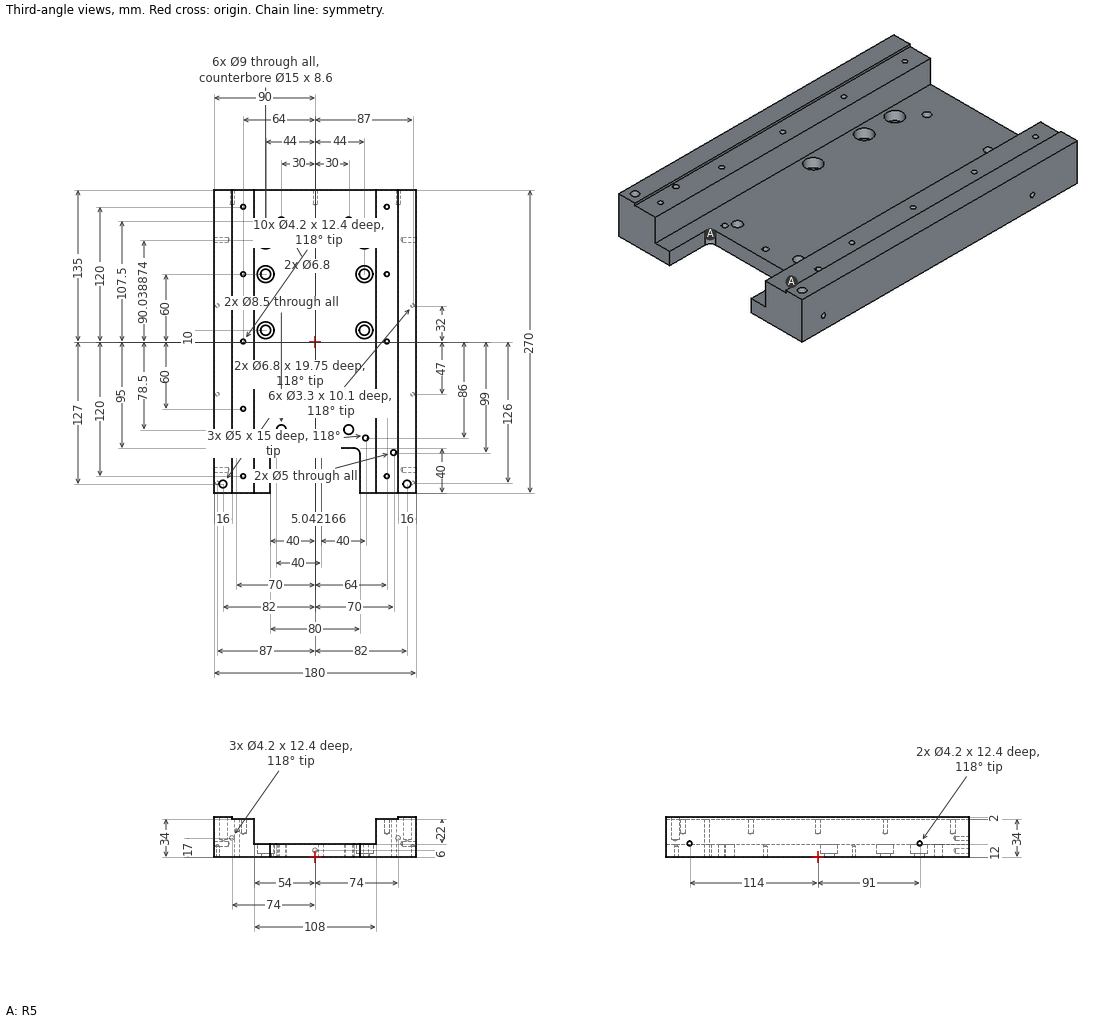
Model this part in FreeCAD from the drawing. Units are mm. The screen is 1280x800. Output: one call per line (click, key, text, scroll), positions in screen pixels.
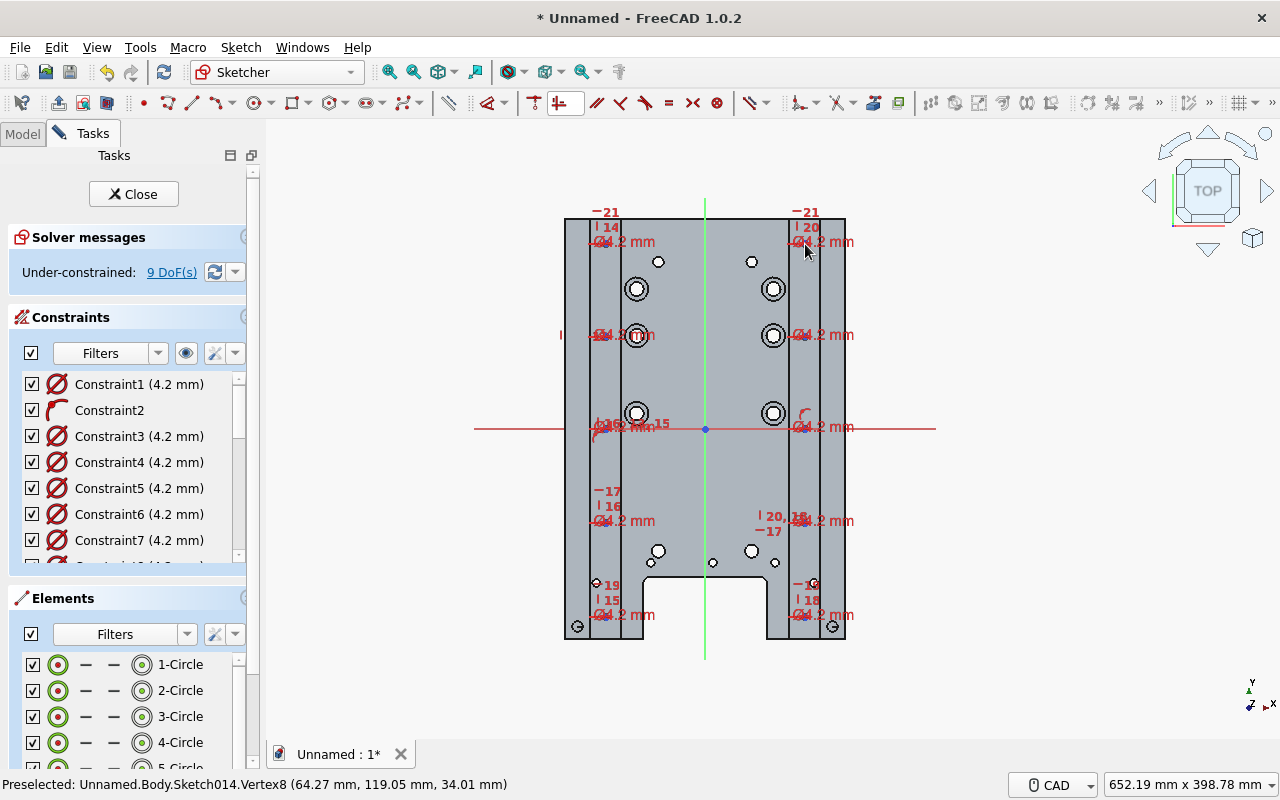
click(805, 244)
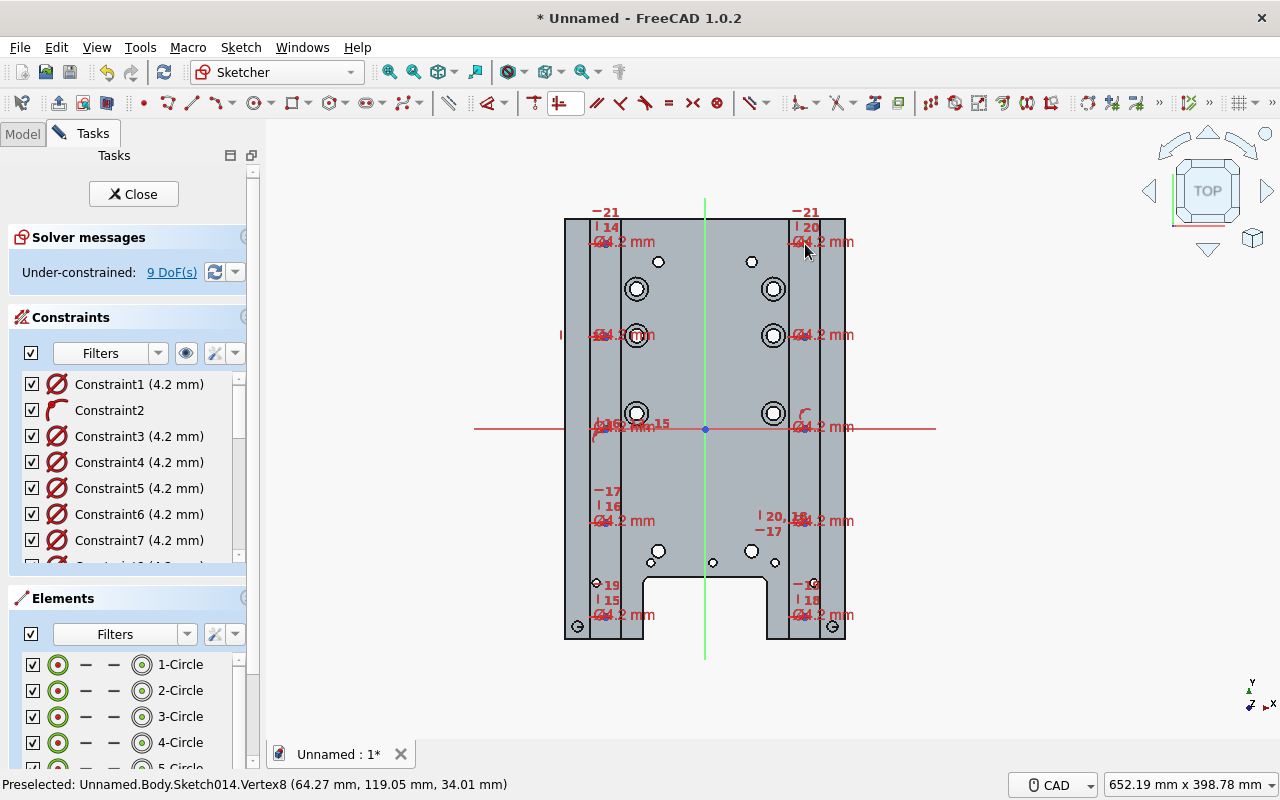
click(805, 337)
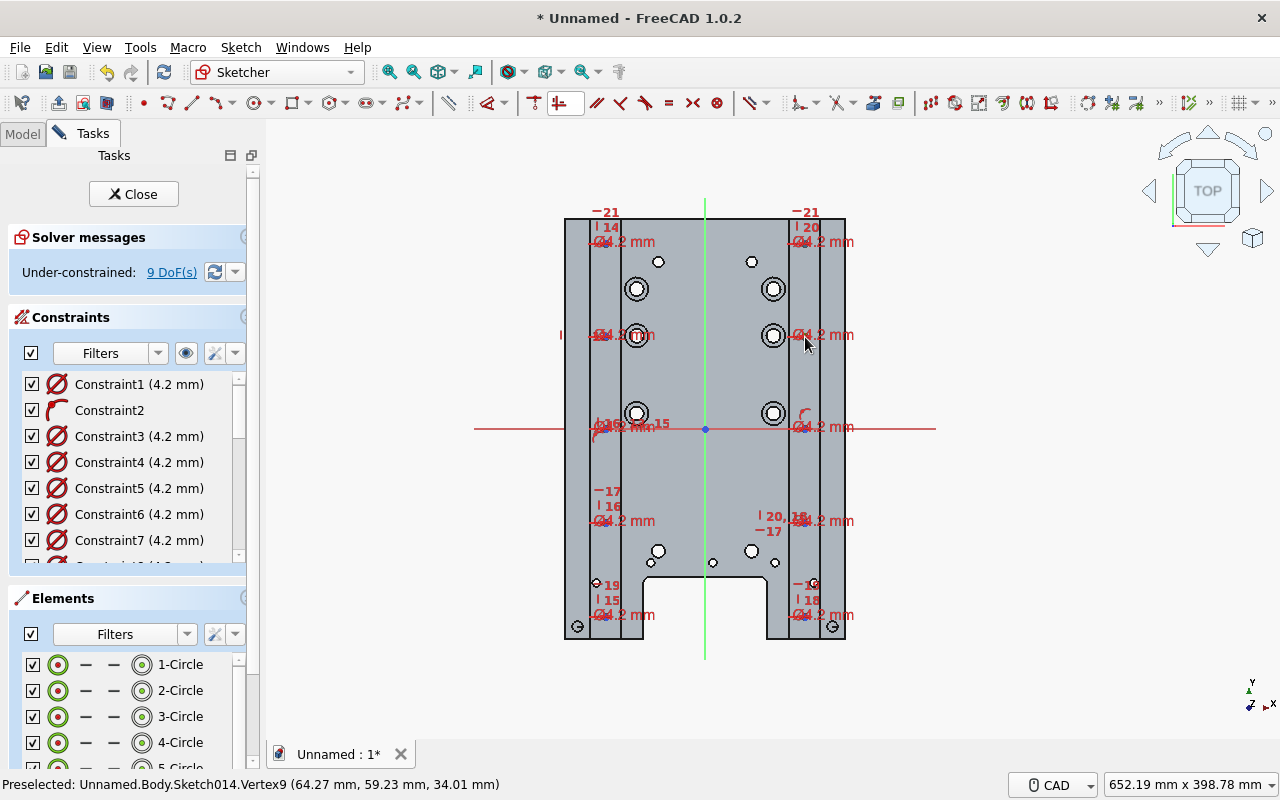
key(v)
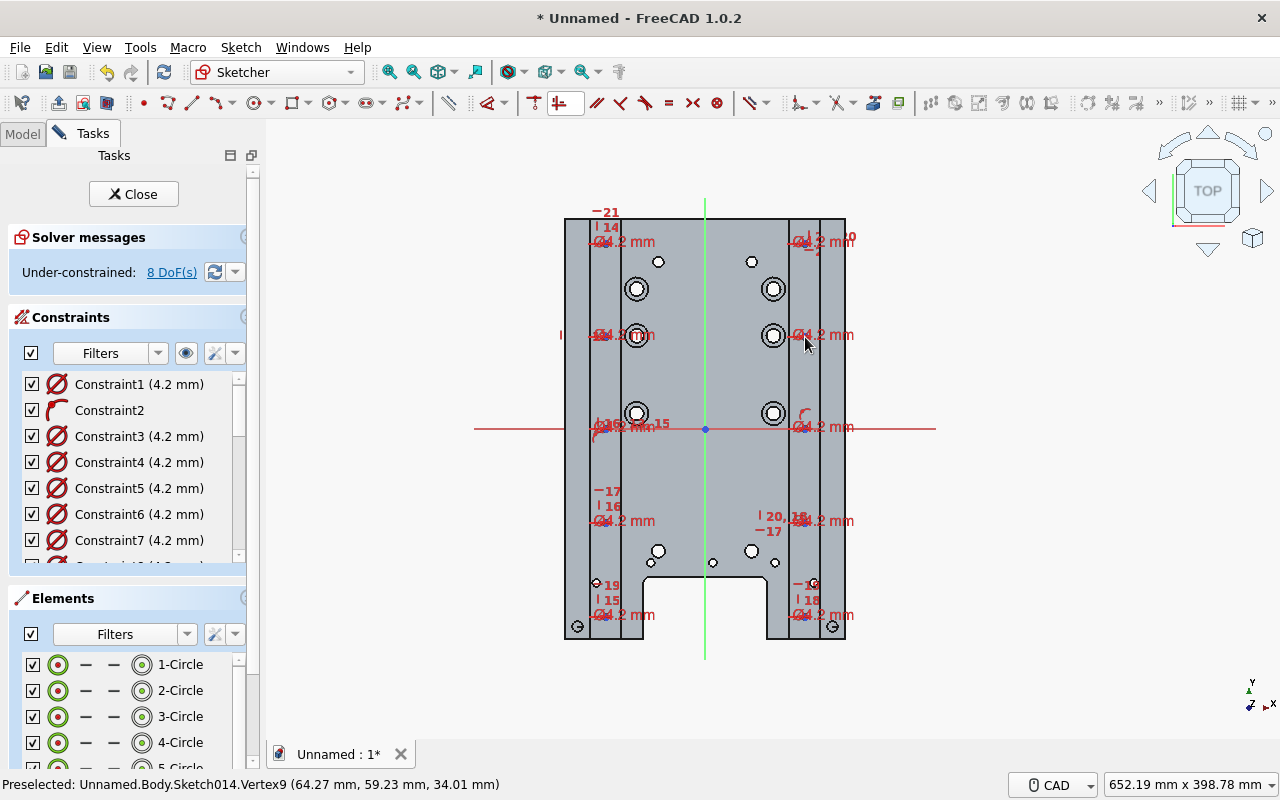
click(606, 337)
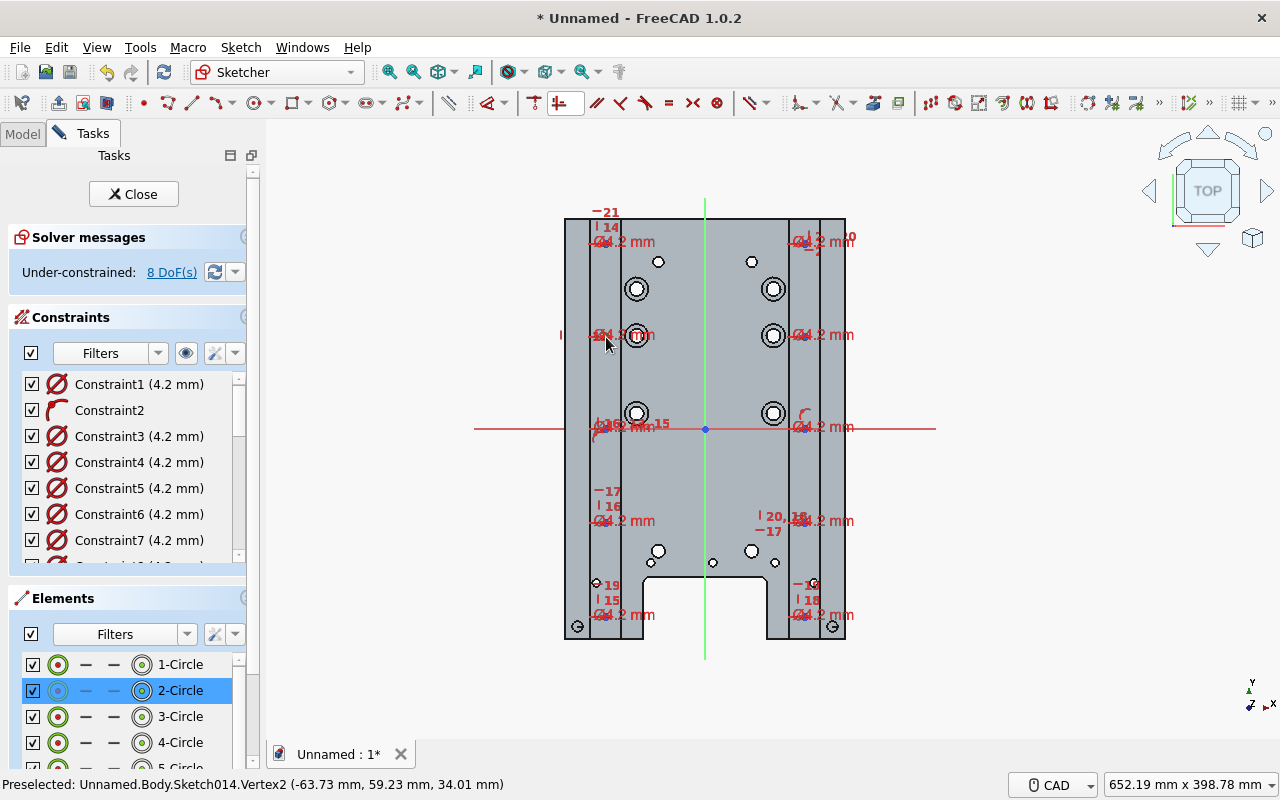
click(805, 337)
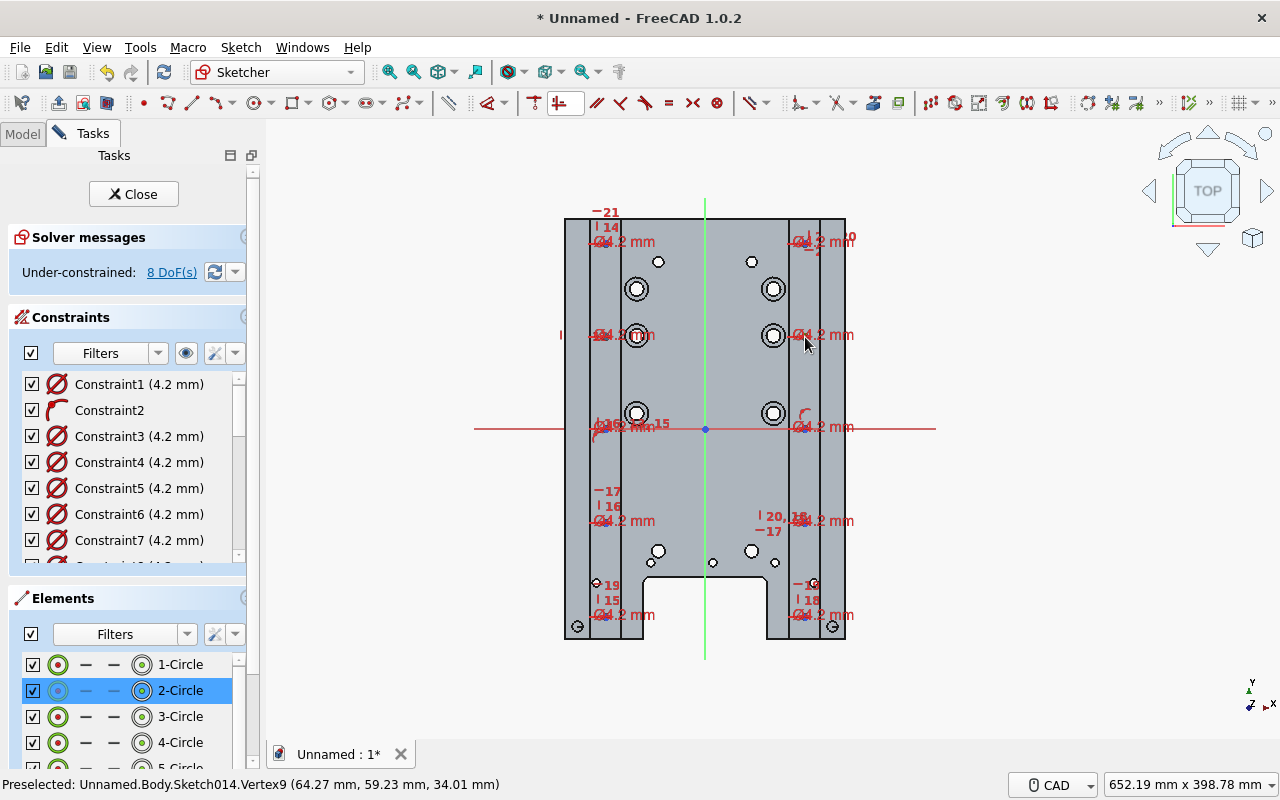
key(h)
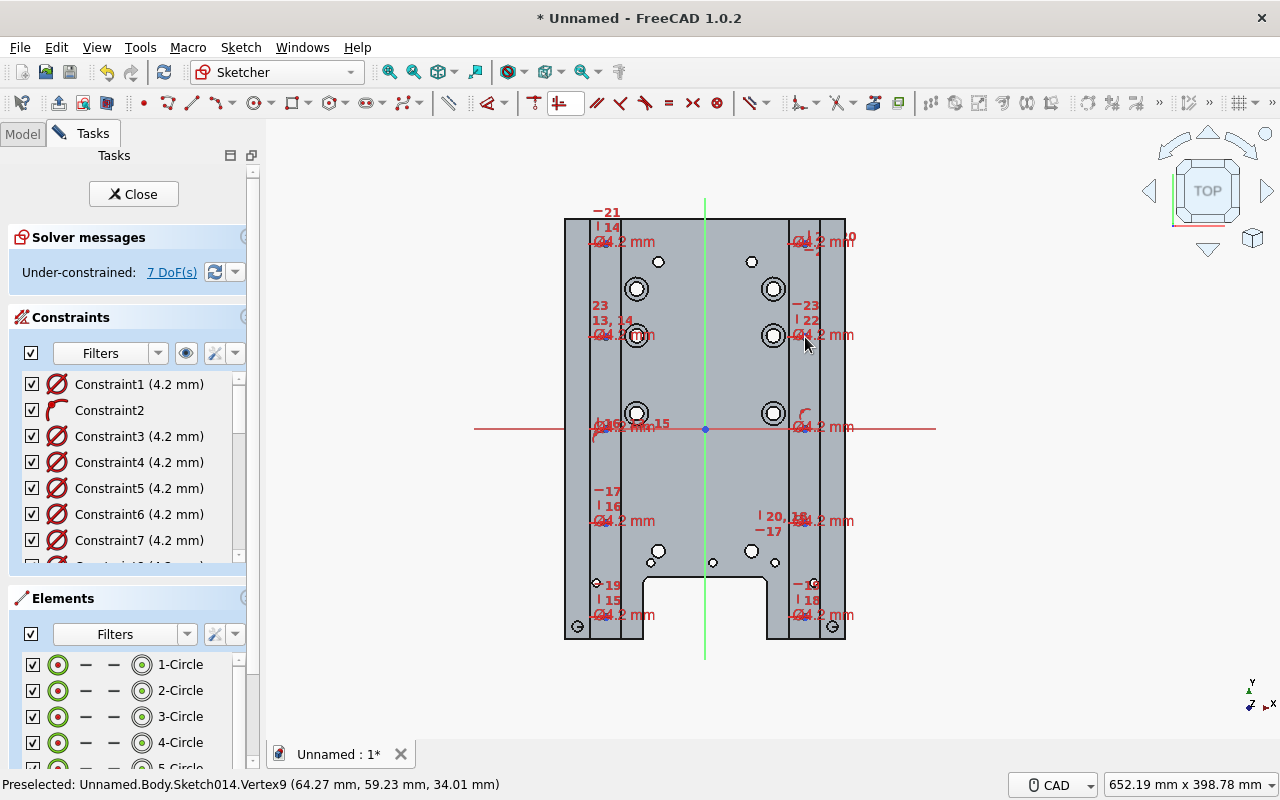
click(805, 523)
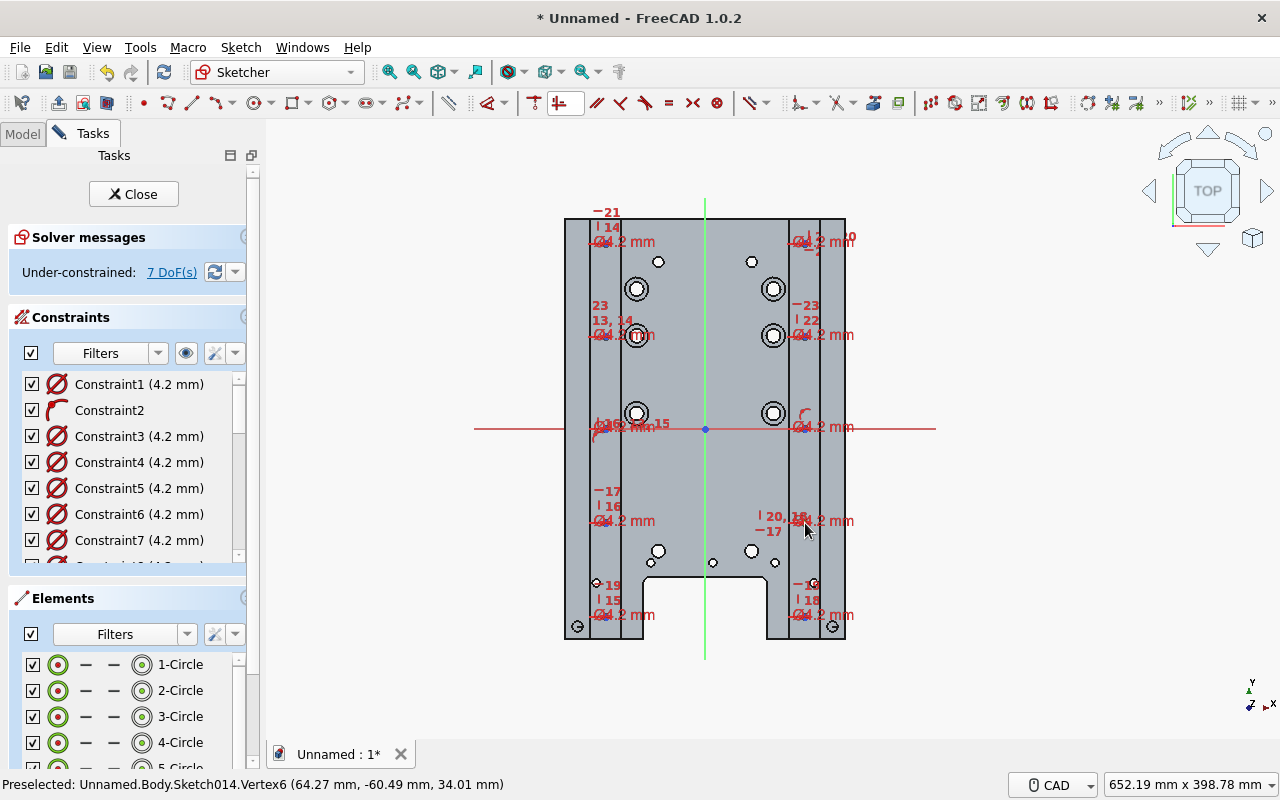
click(805, 429)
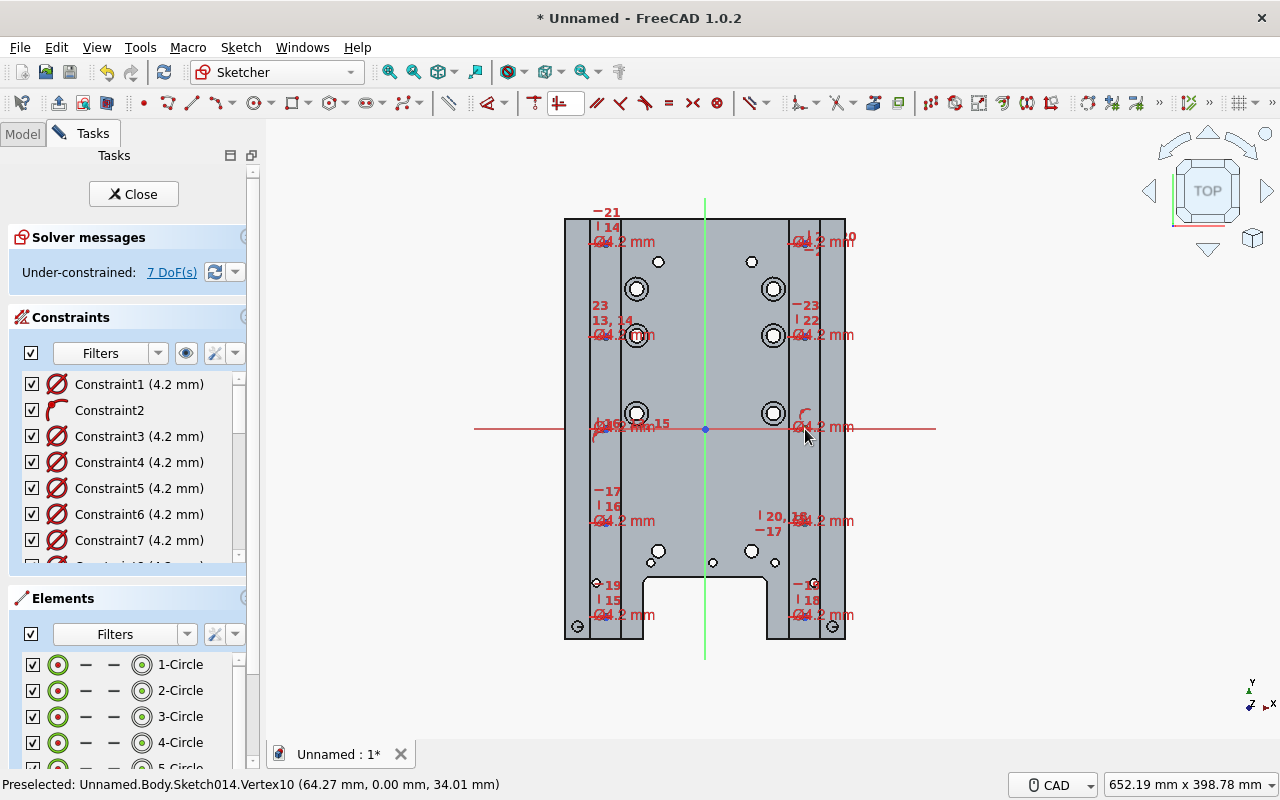
key(v)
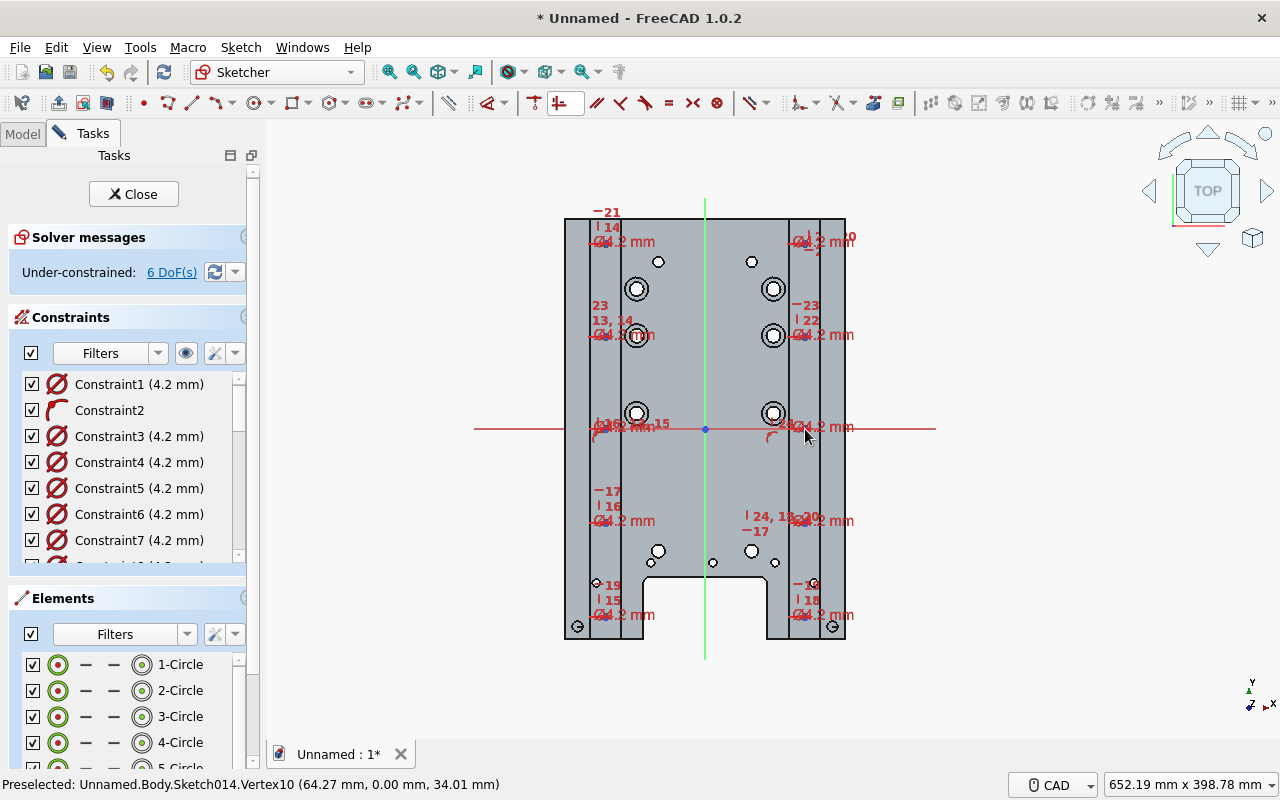
click(488, 104)